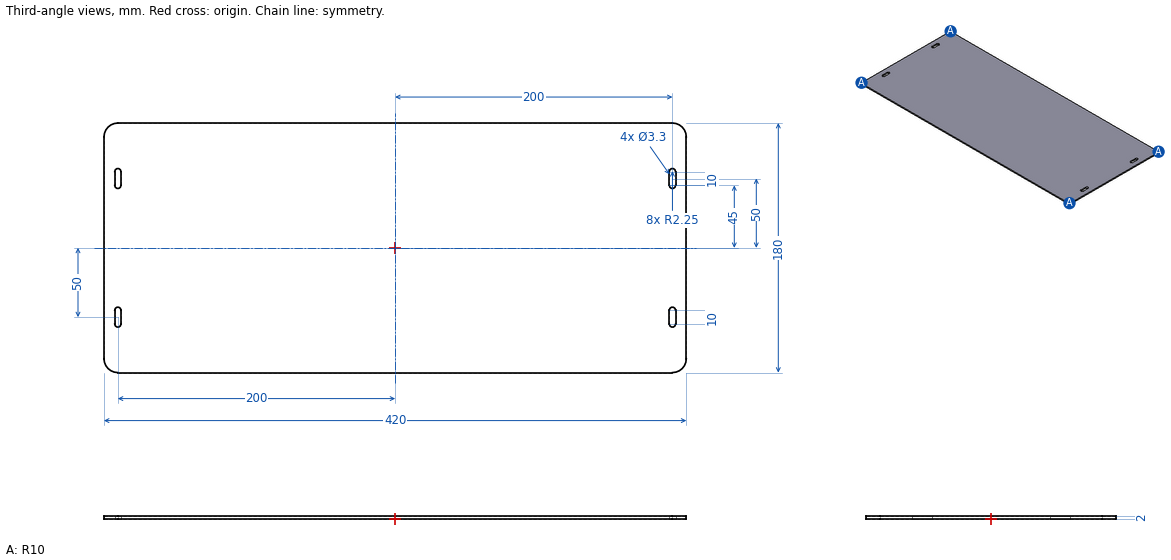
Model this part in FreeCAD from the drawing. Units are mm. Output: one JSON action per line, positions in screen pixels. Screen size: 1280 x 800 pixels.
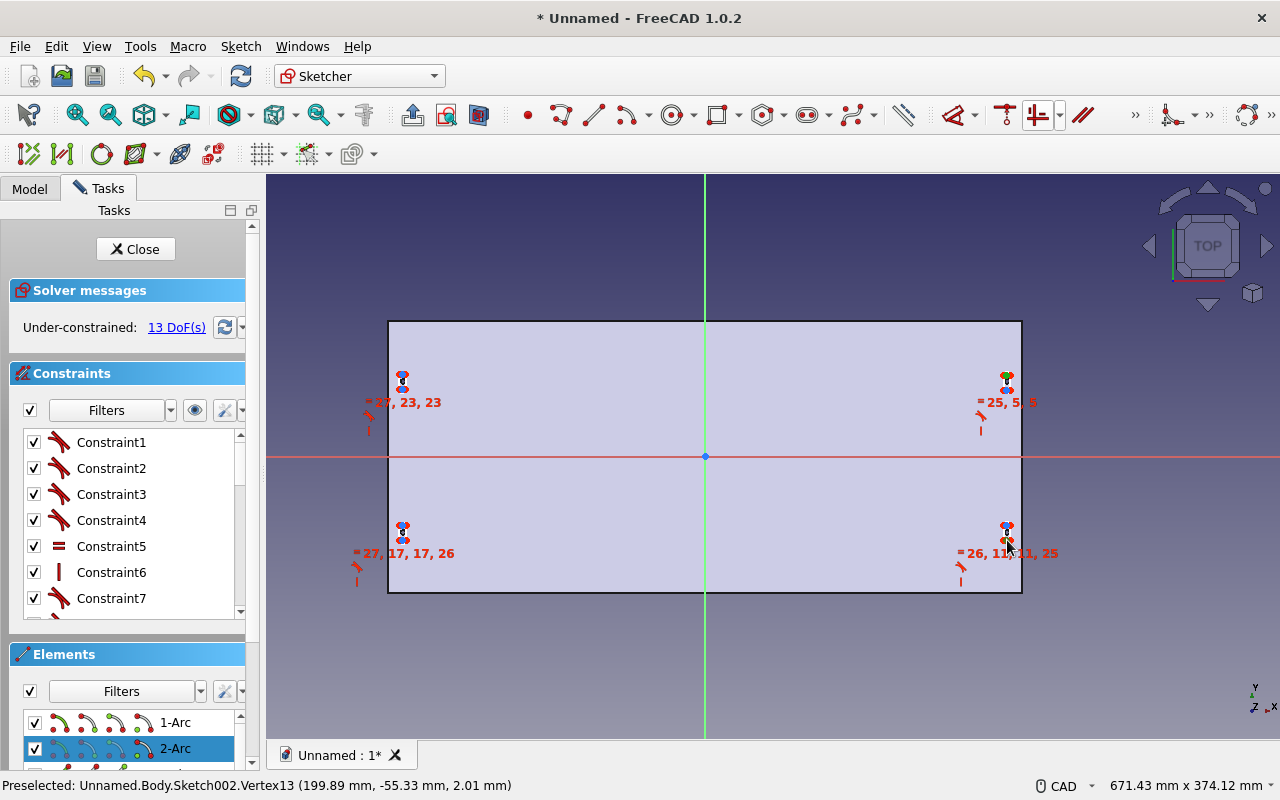
{"action": "left_click", "coordinate": [353, 457]}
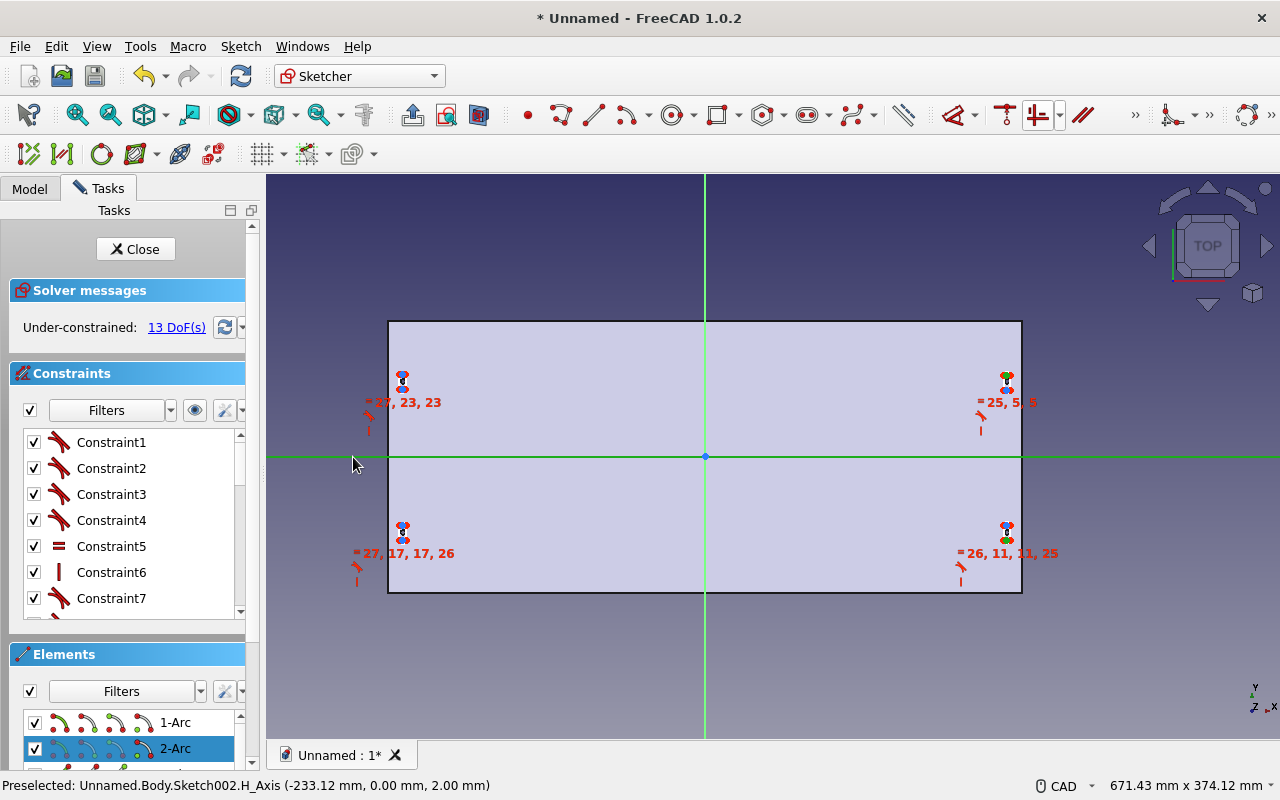
{"action": "key", "text": "s"}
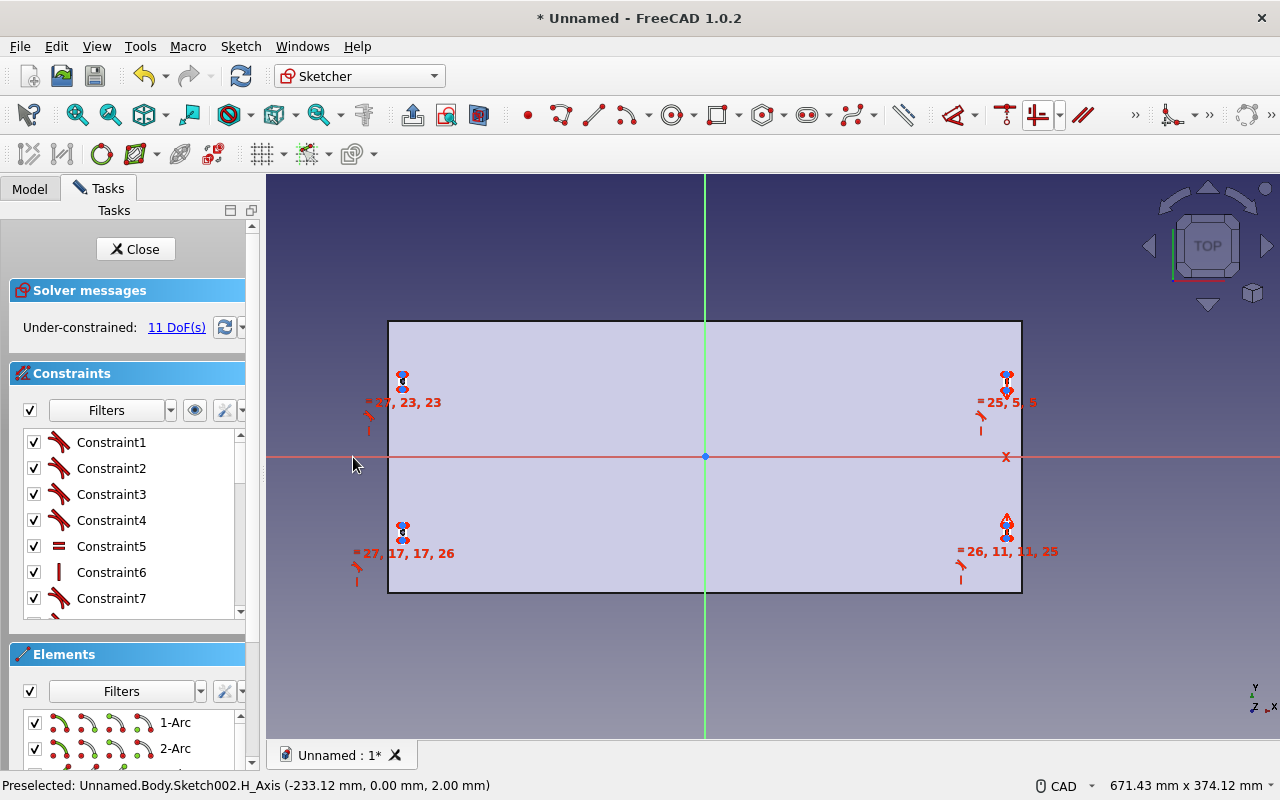
{"action": "scroll", "coordinate": [1007, 538], "scroll_direction": "up", "scroll_amount": 7}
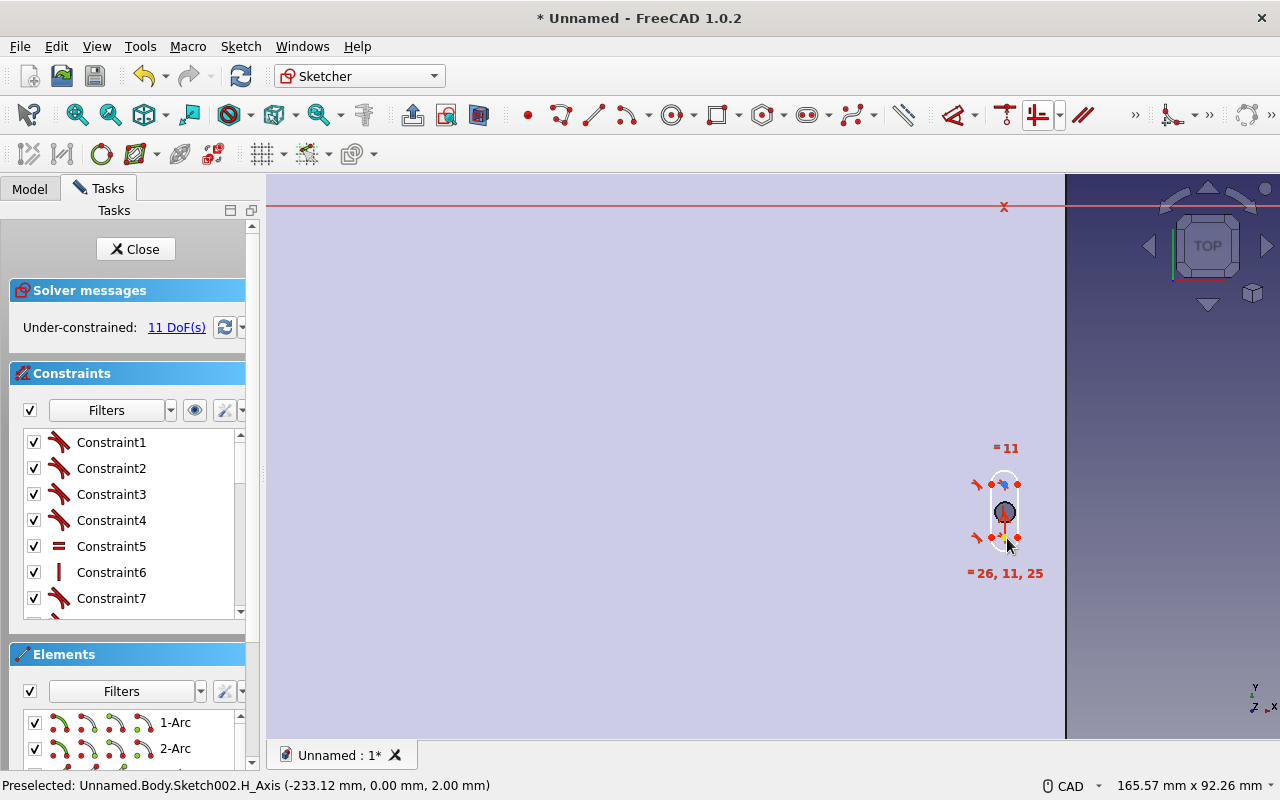
{"action": "left_click", "coordinate": [1005, 538]}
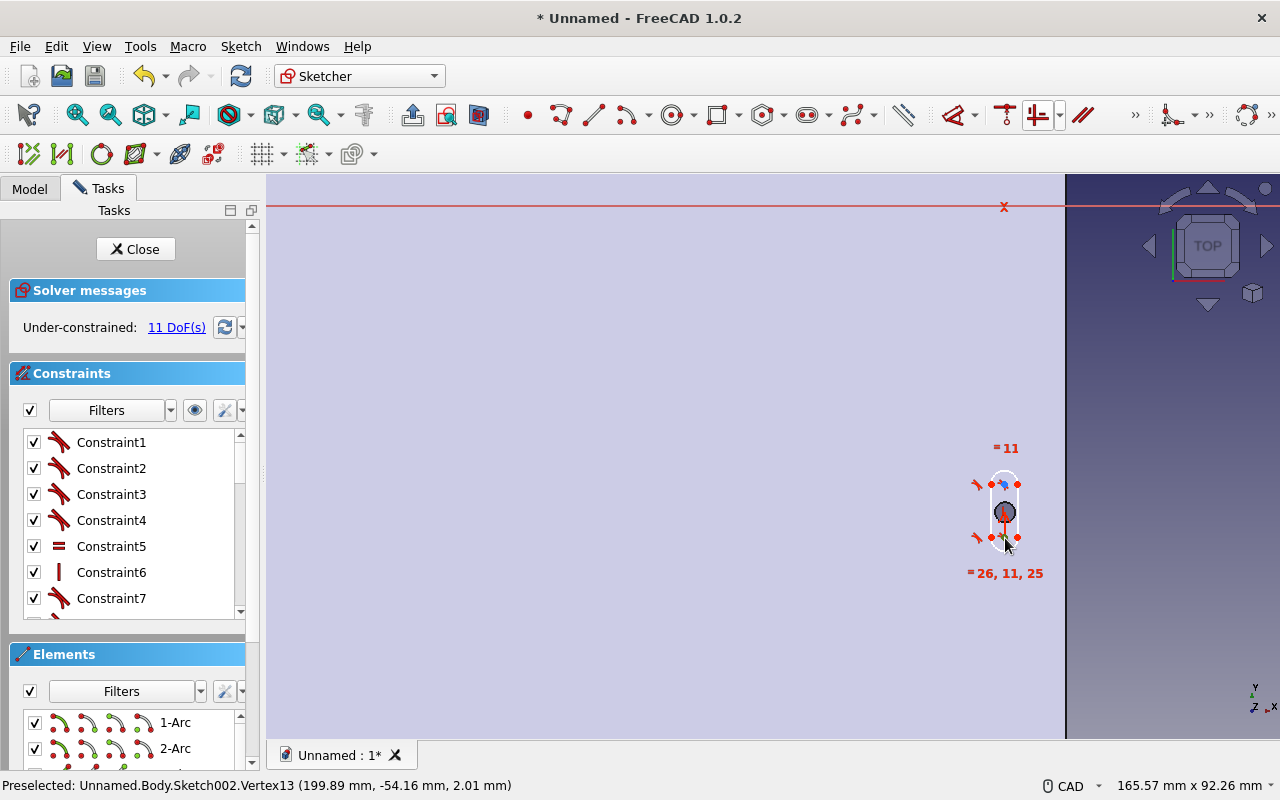
{"action": "scroll", "coordinate": [1007, 538], "scroll_direction": "down", "scroll_amount": 7}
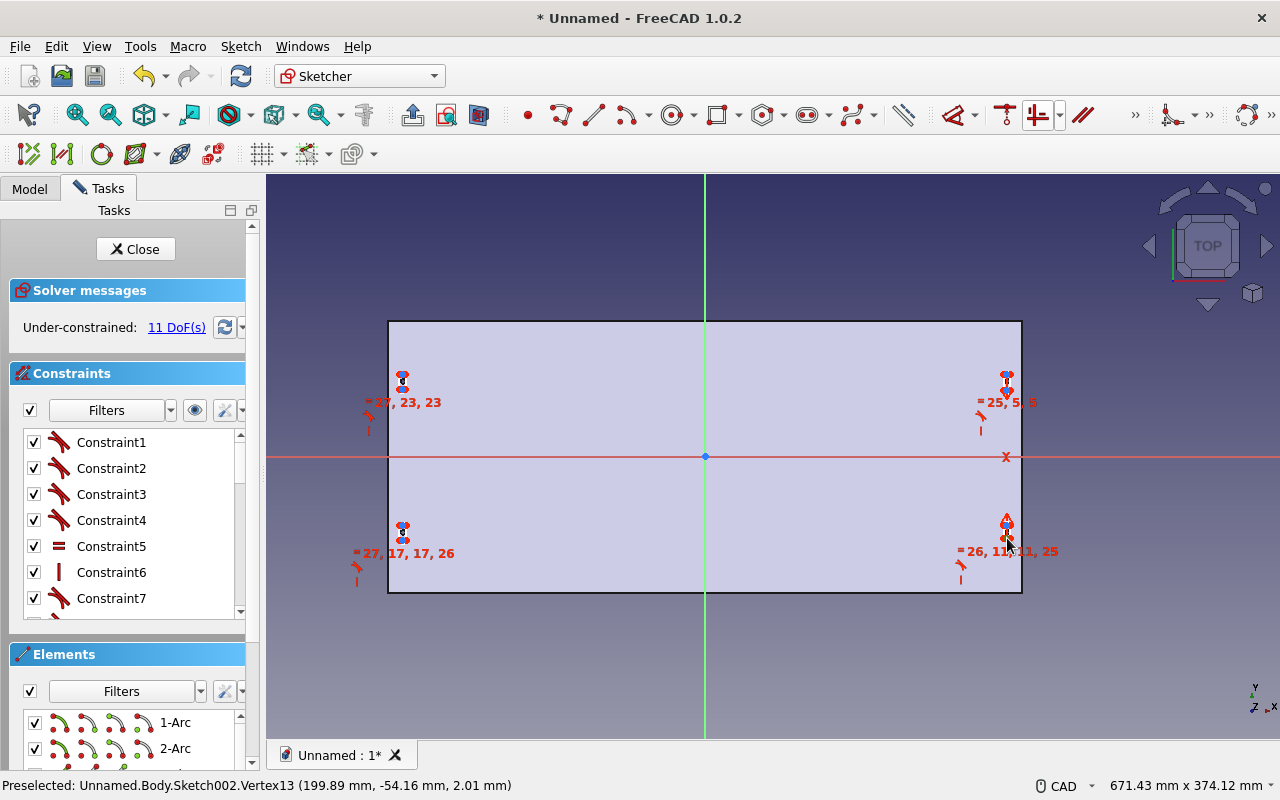
{"action": "scroll", "coordinate": [403, 541], "scroll_direction": "up", "scroll_amount": 7}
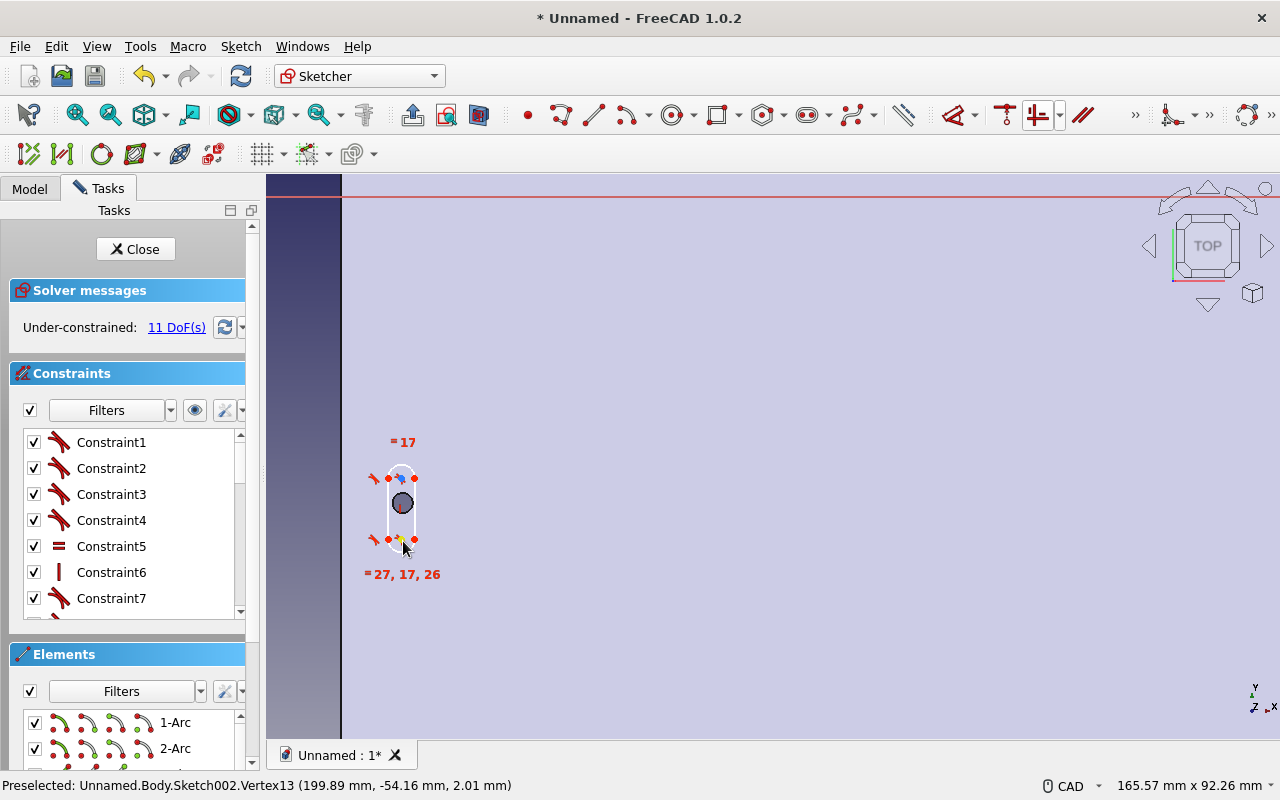
{"action": "left_click", "coordinate": [402, 539]}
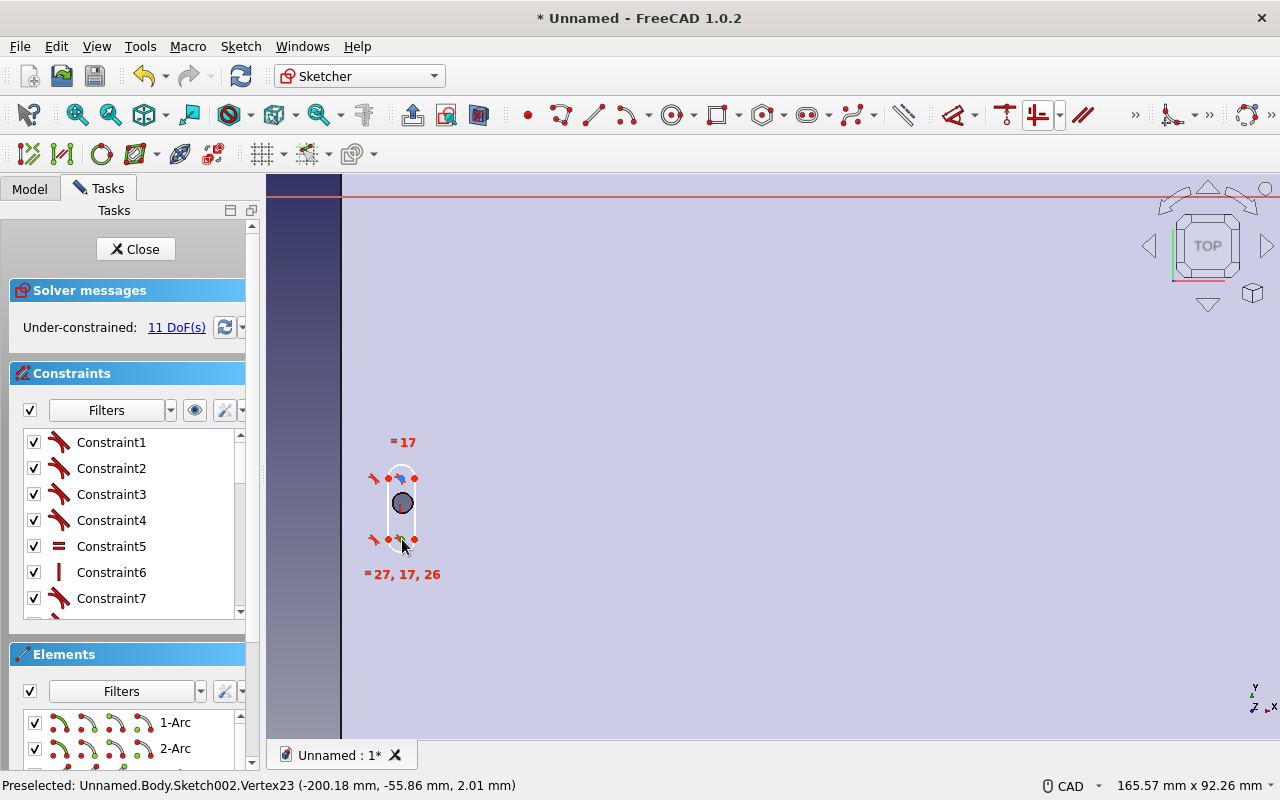
{"action": "scroll", "coordinate": [402, 541], "scroll_direction": "down", "scroll_amount": 7}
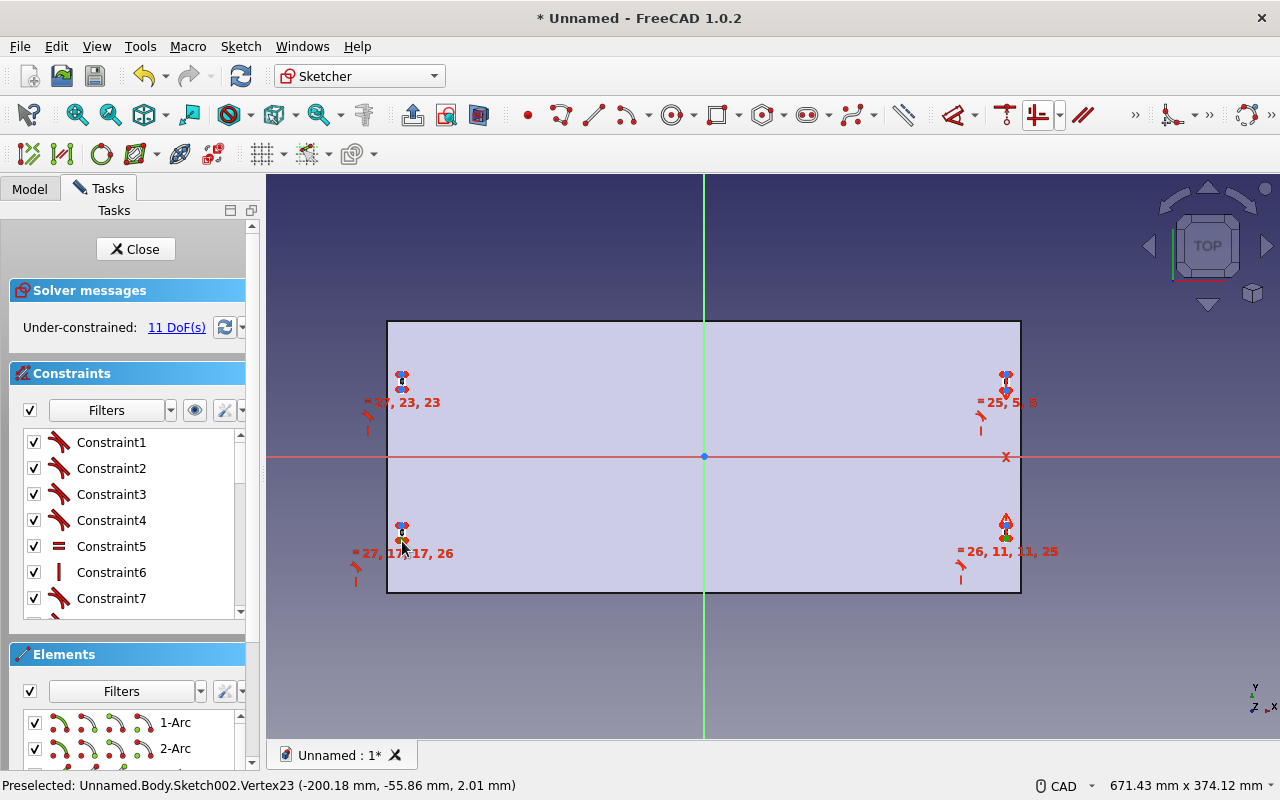
{"action": "left_click", "coordinate": [704, 675]}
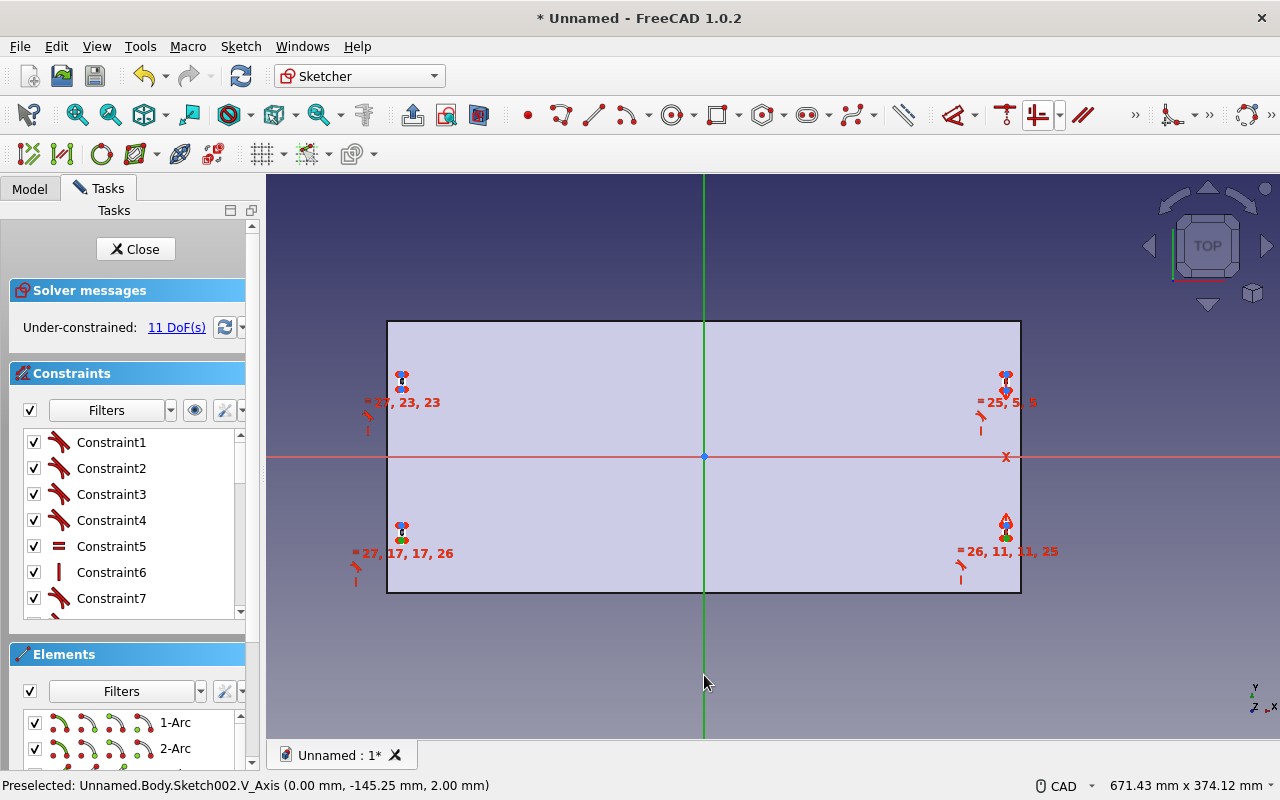
{"action": "key", "text": "s"}